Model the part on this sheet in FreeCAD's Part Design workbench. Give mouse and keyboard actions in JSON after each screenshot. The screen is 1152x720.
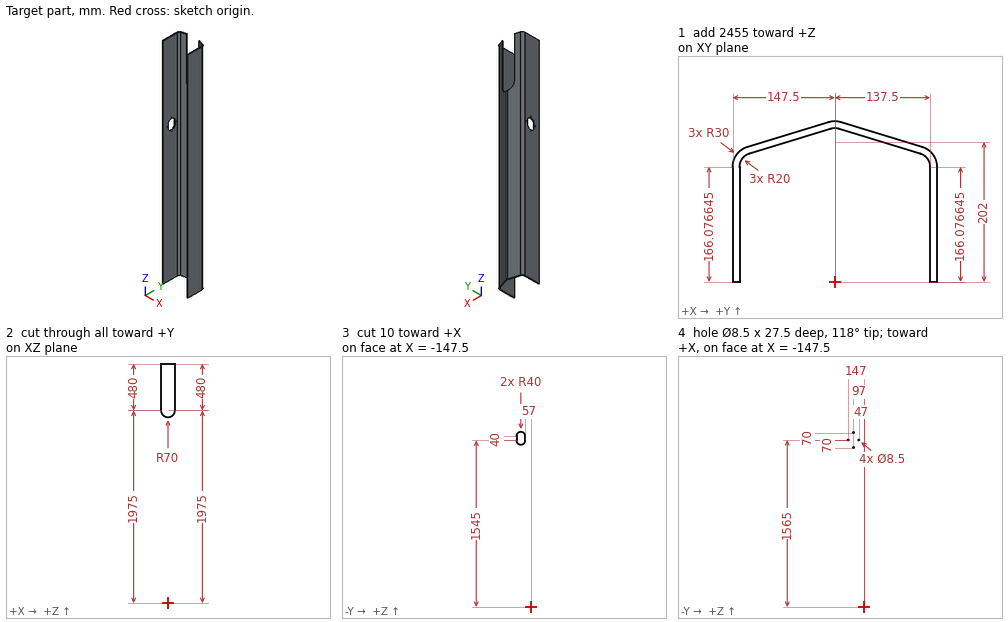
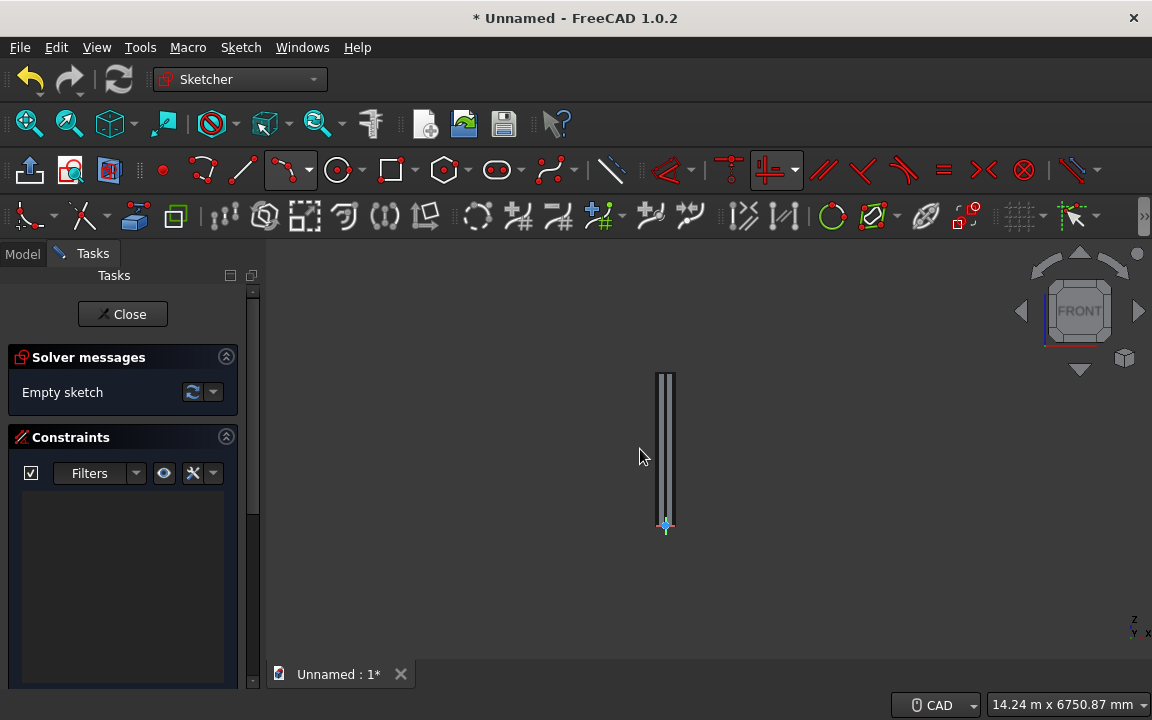
{"action": "scroll", "coordinate": [670, 381], "scroll_direction": "up", "scroll_amount": 10}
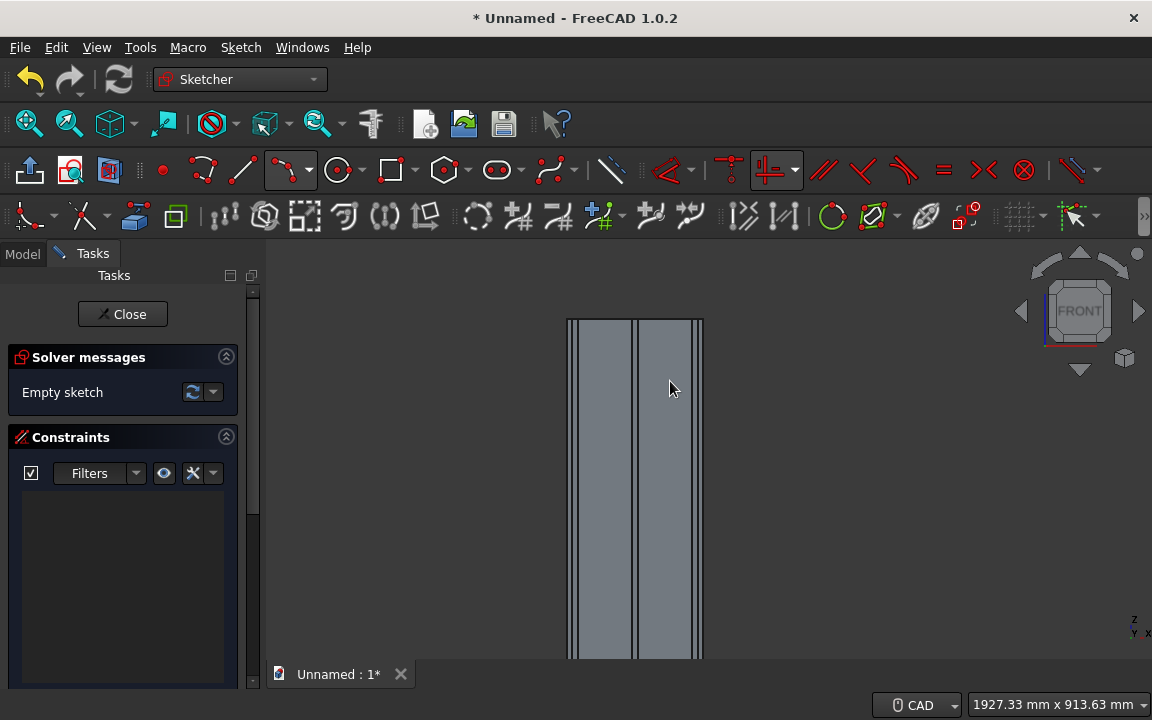
{"action": "left_click", "coordinate": [204, 170]}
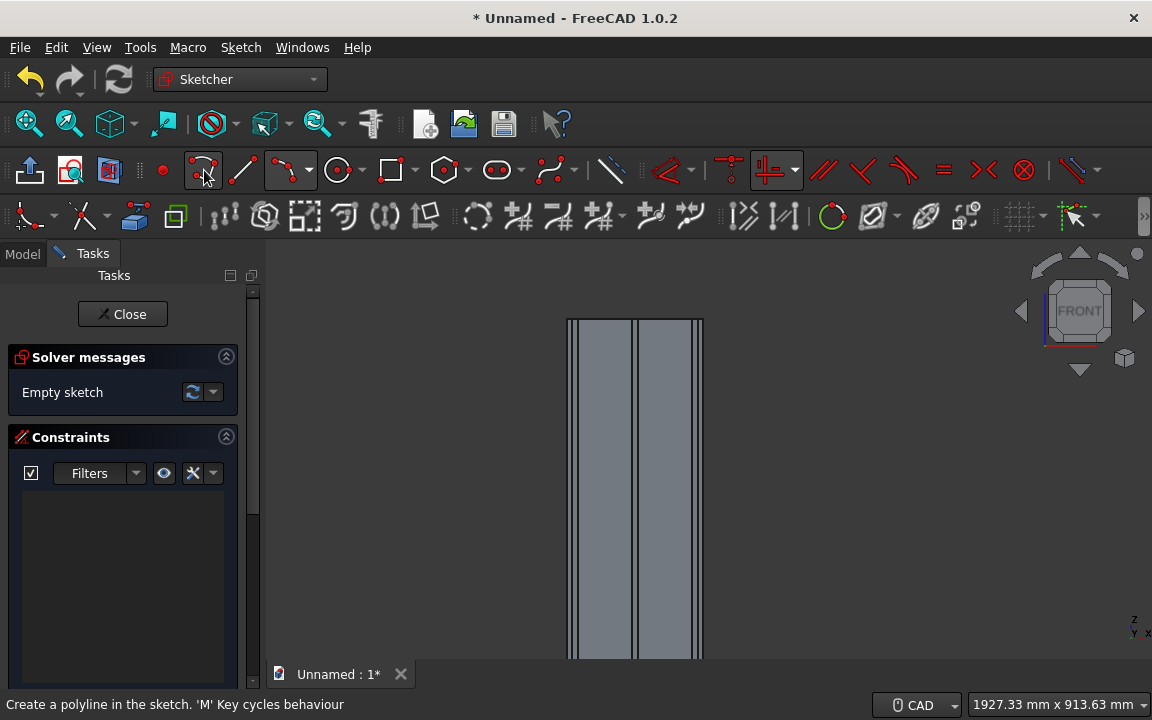
{"action": "left_click", "coordinate": [603, 540]}
{"action": "left_click", "coordinate": [603, 319]}
{"action": "left_click", "coordinate": [667, 319]}
{"action": "left_click", "coordinate": [667, 540]}
{"action": "right_click", "coordinate": [667, 540]}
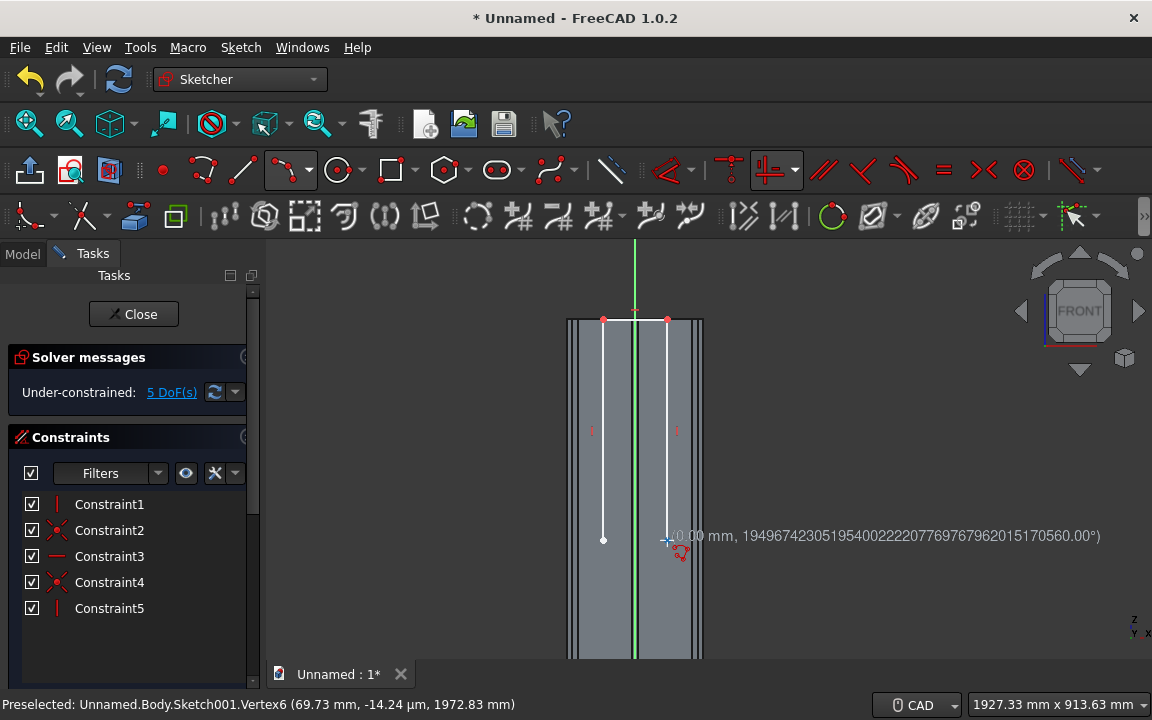
{"action": "left_click", "coordinate": [284, 170]}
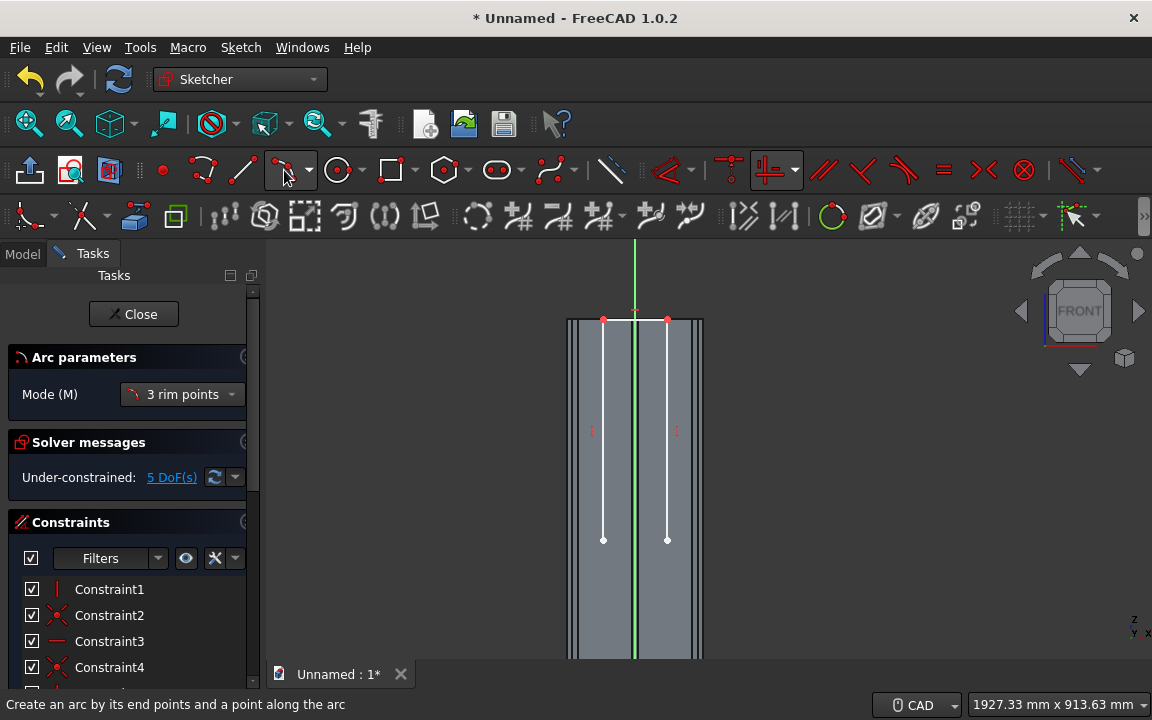
{"action": "left_click", "coordinate": [667, 541]}
{"action": "left_click", "coordinate": [603, 541]}
{"action": "left_click", "coordinate": [616, 566]}
{"action": "key", "text": "Escape"}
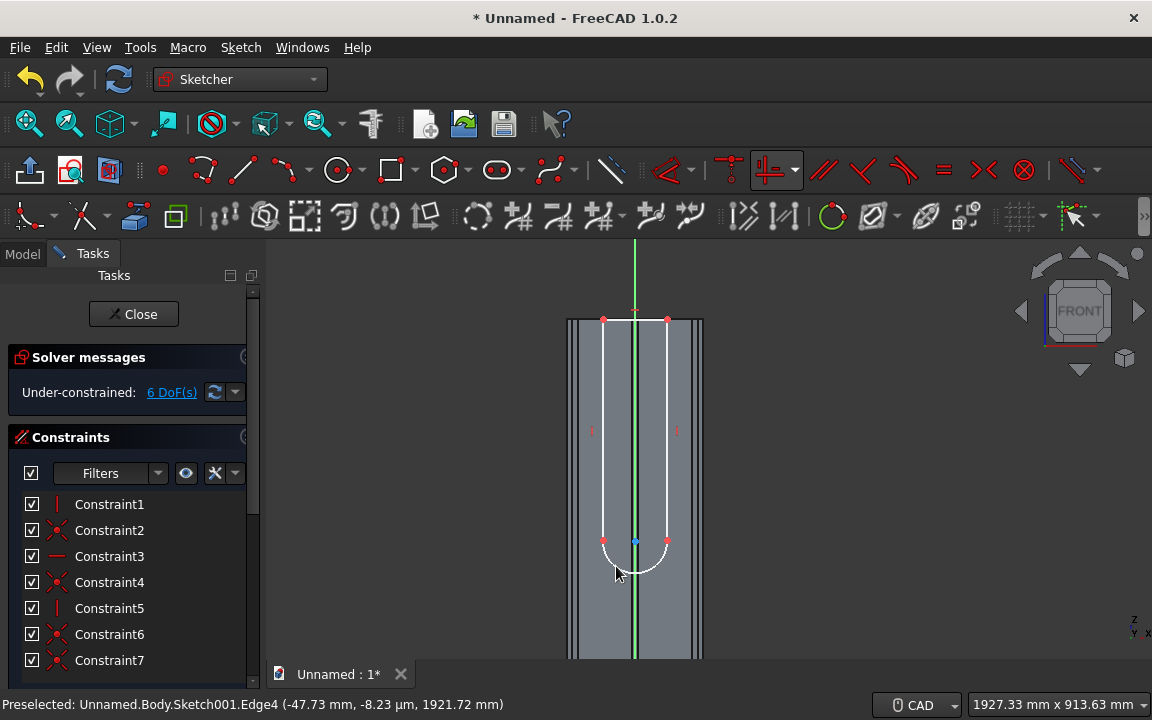
{"action": "left_click", "coordinate": [635, 541]}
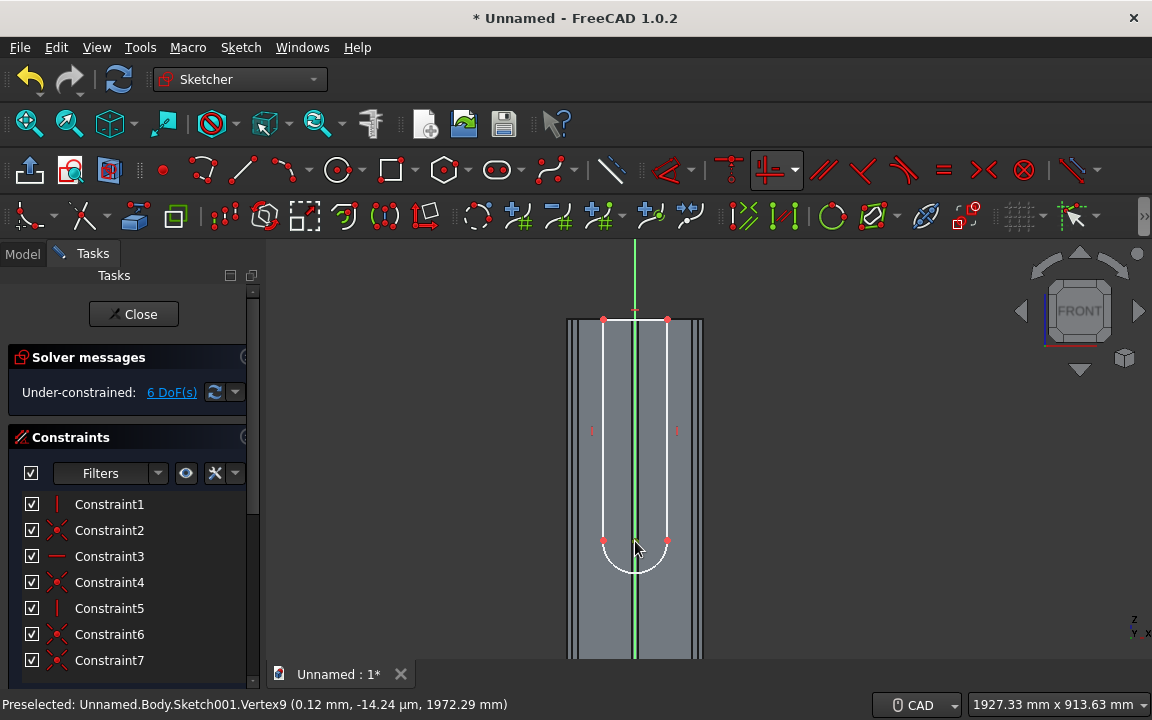
{"action": "left_click", "coordinate": [635, 605]}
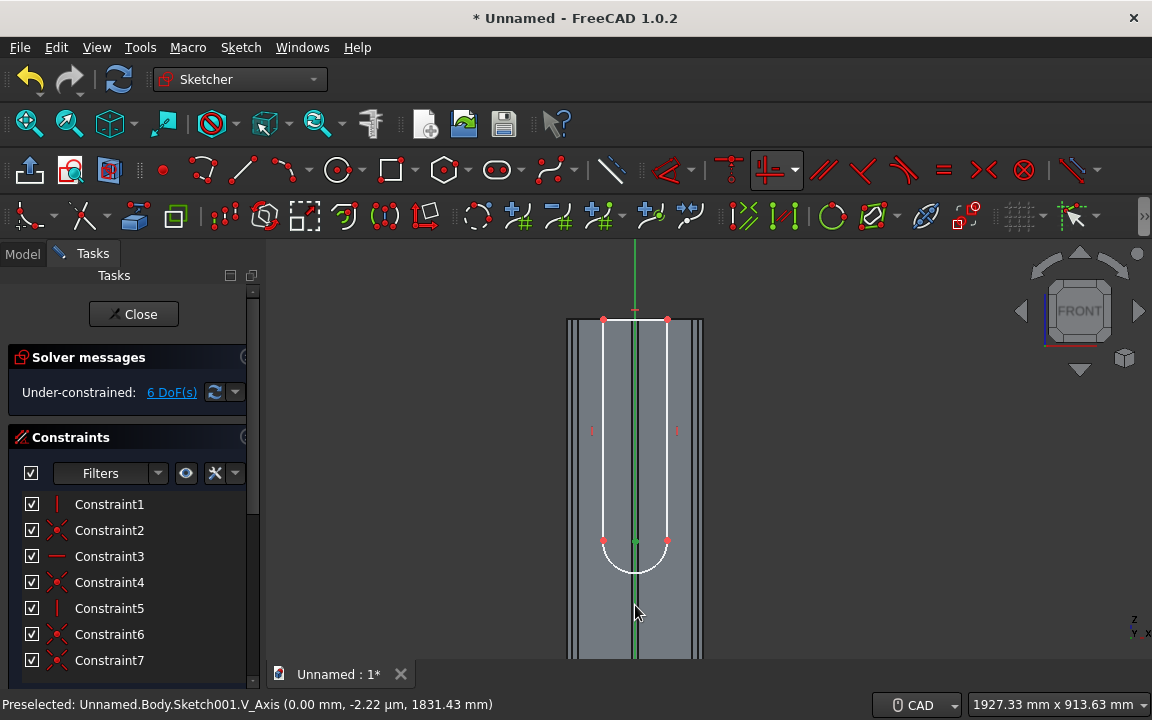
{"action": "left_click", "coordinate": [730, 170]}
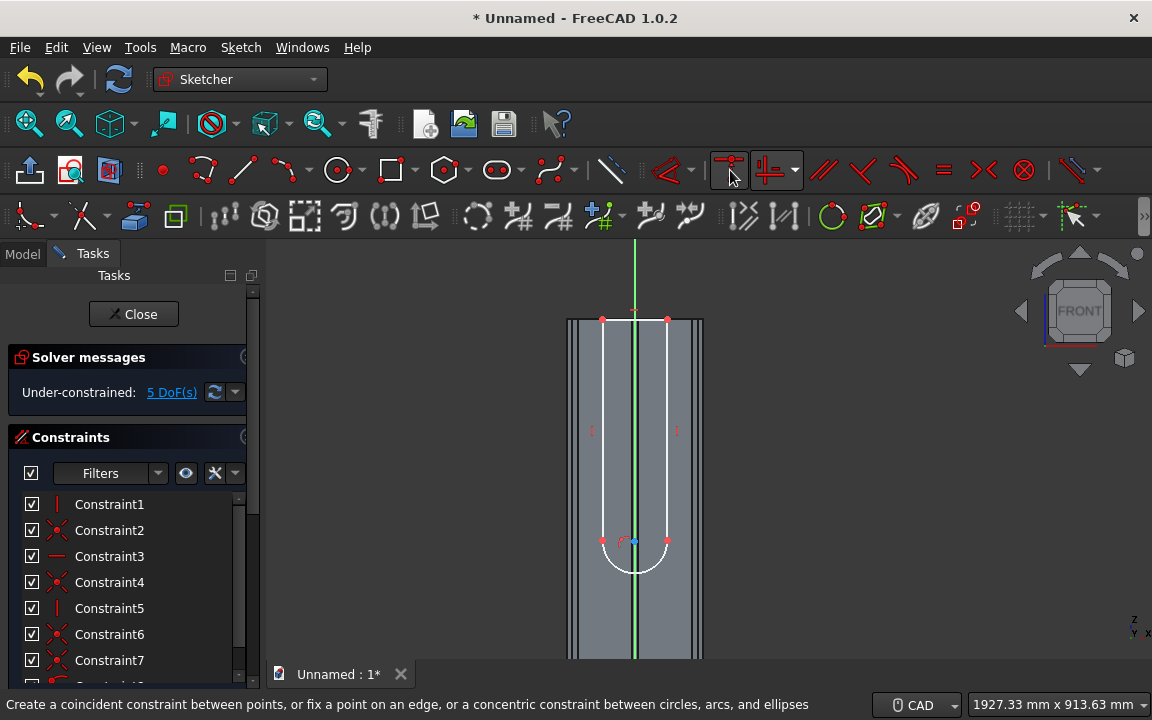
{"action": "left_click", "coordinate": [666, 170]}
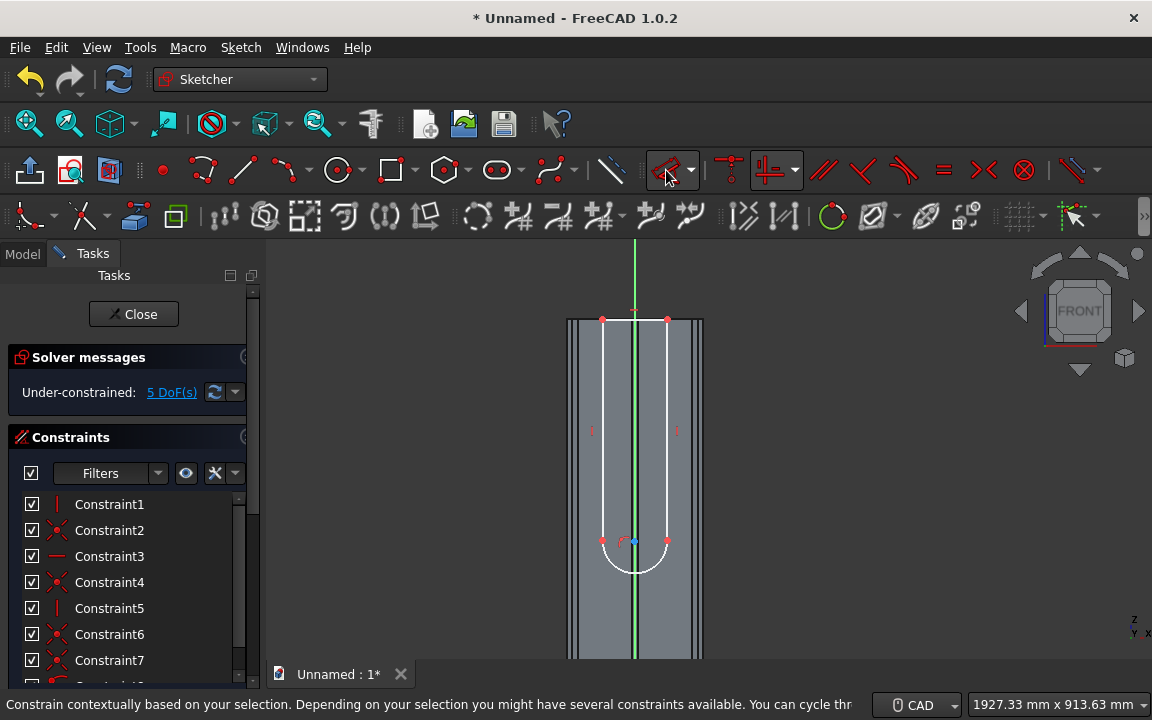
{"action": "scroll", "coordinate": [616, 567], "scroll_direction": "up", "scroll_amount": 2}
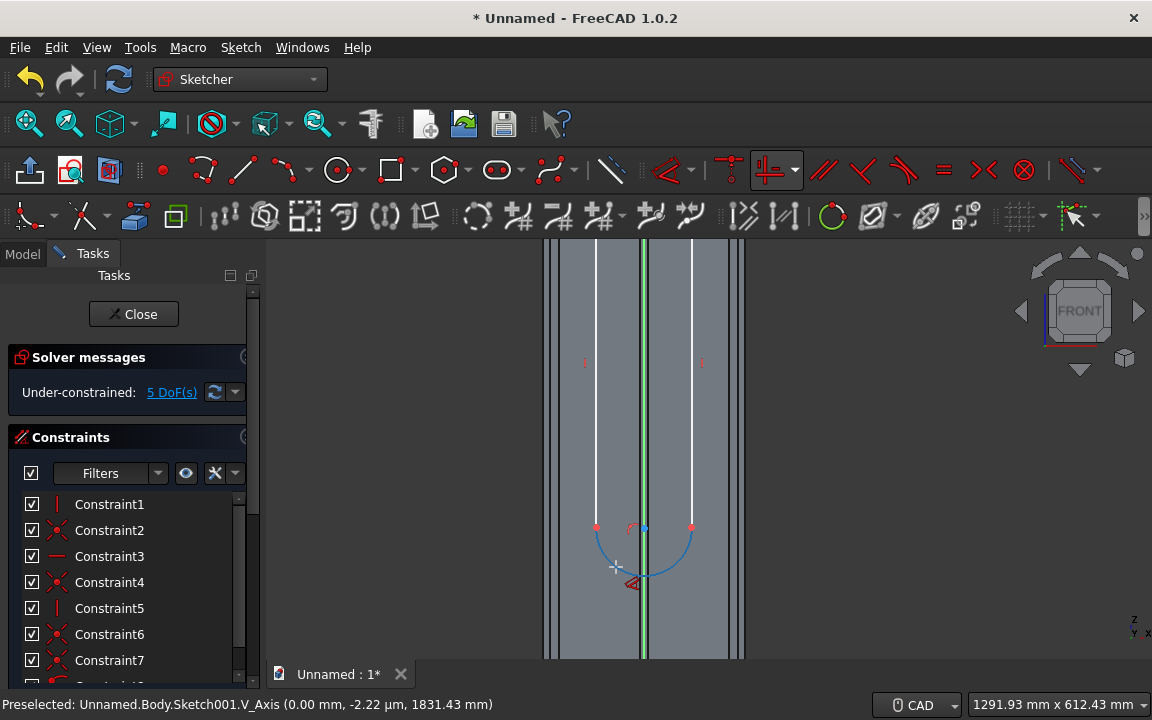
{"action": "left_click", "coordinate": [616, 567]}
{"action": "left_click", "coordinate": [597, 593]}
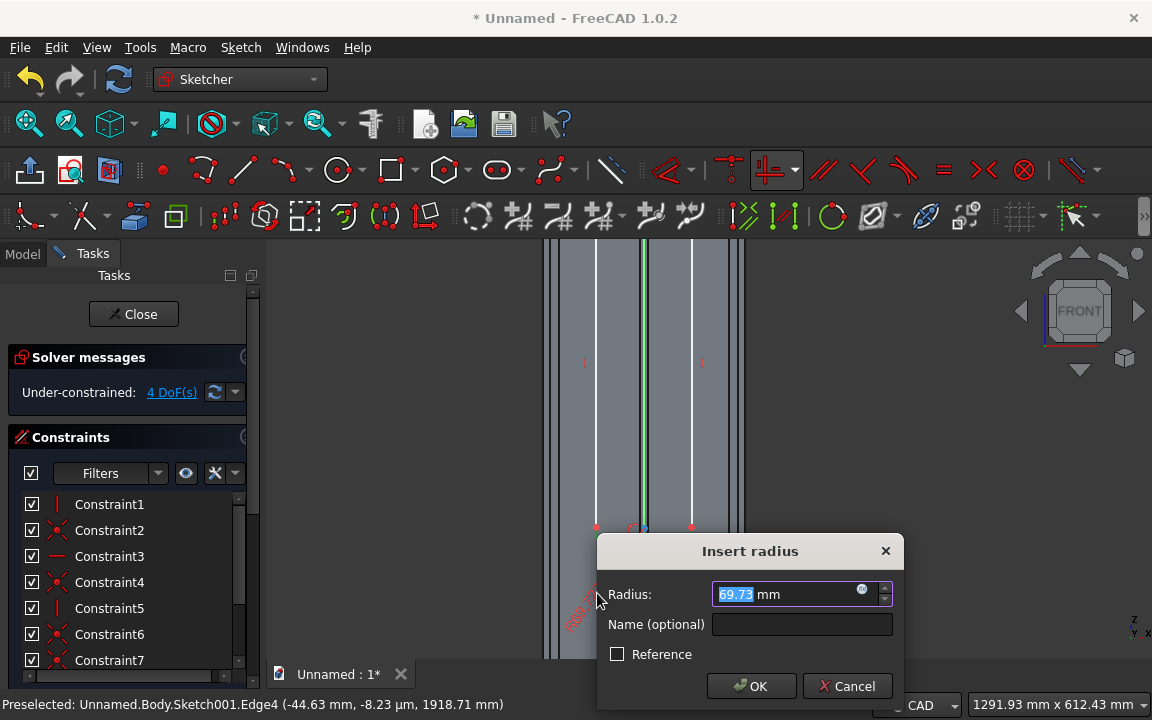
{"action": "type", "text": "70"}
{"action": "key", "text": "Return"}